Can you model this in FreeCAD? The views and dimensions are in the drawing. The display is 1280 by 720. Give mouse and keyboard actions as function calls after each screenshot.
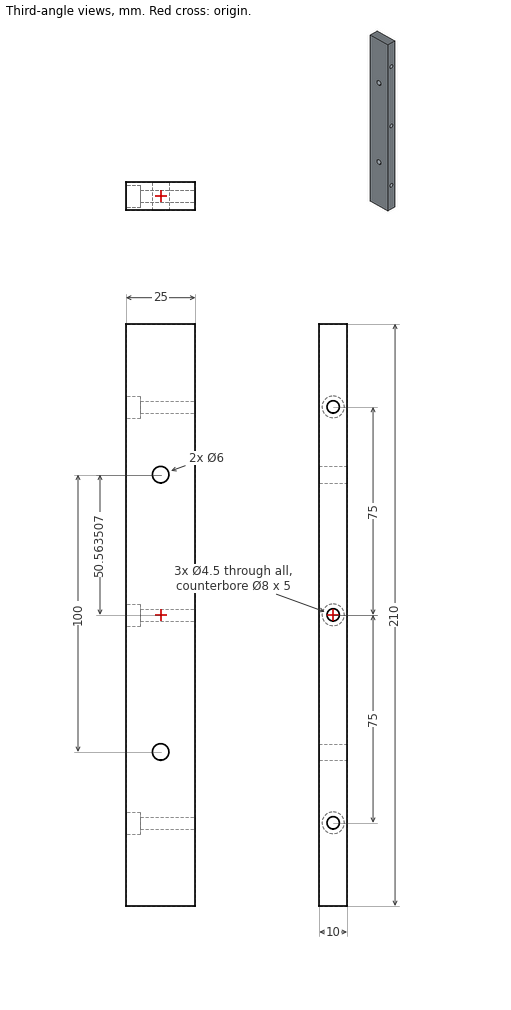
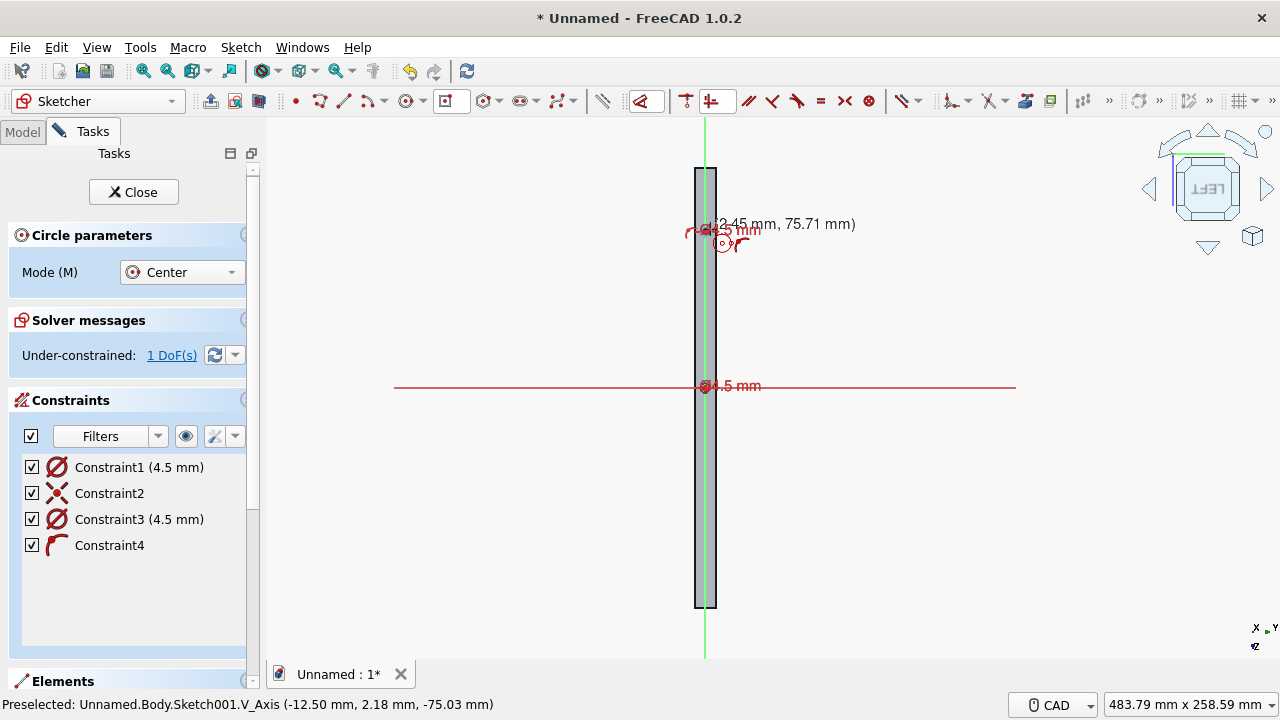
scroll(705, 545, up, 8)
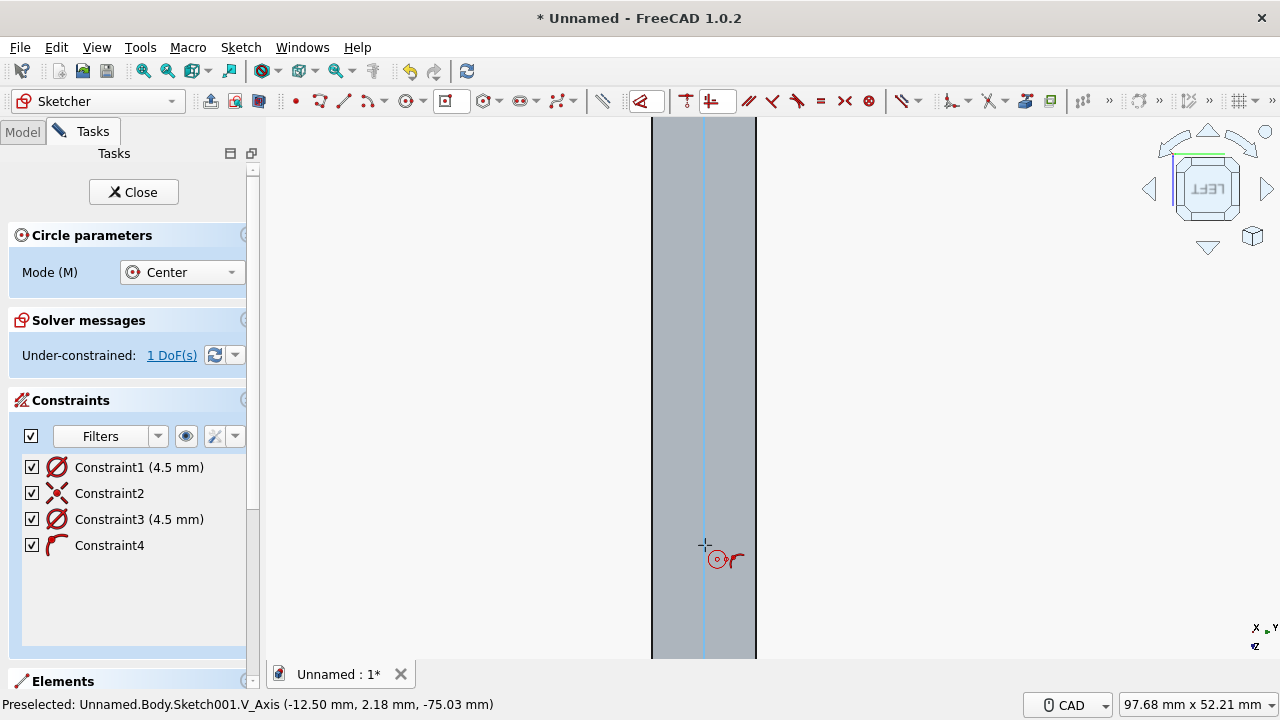
scroll(705, 546, down, 8)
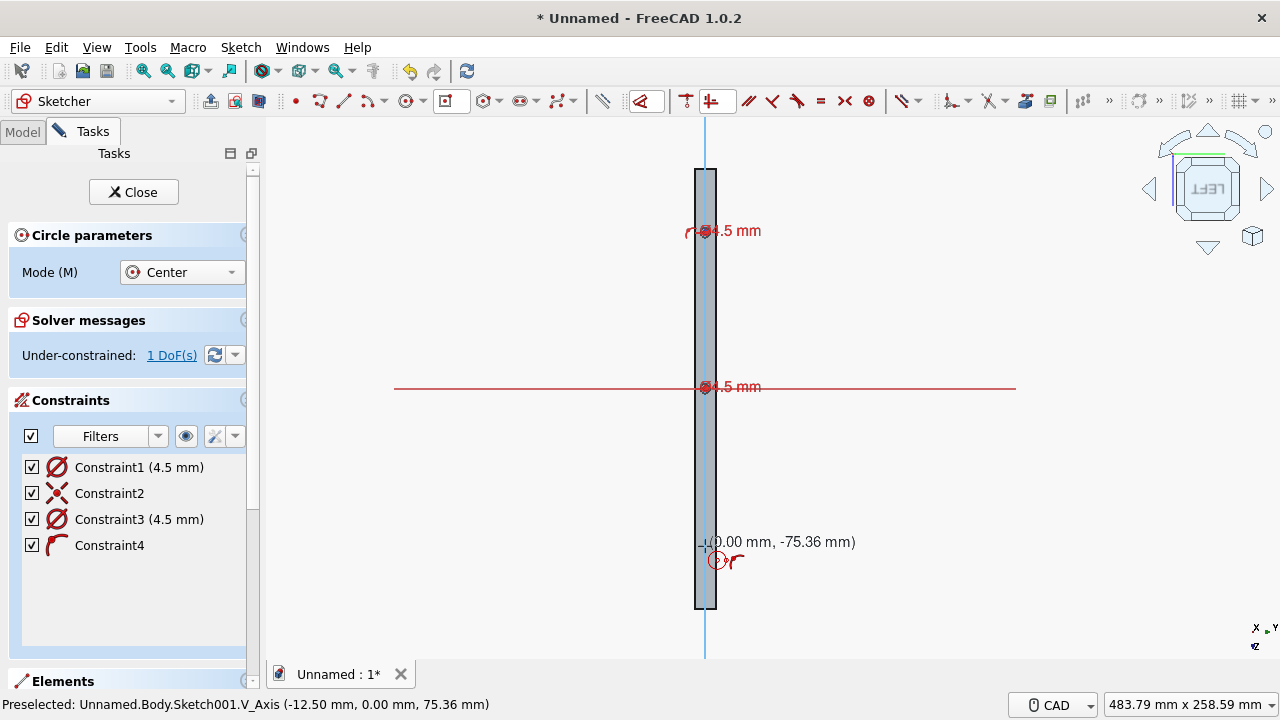
click(705, 546)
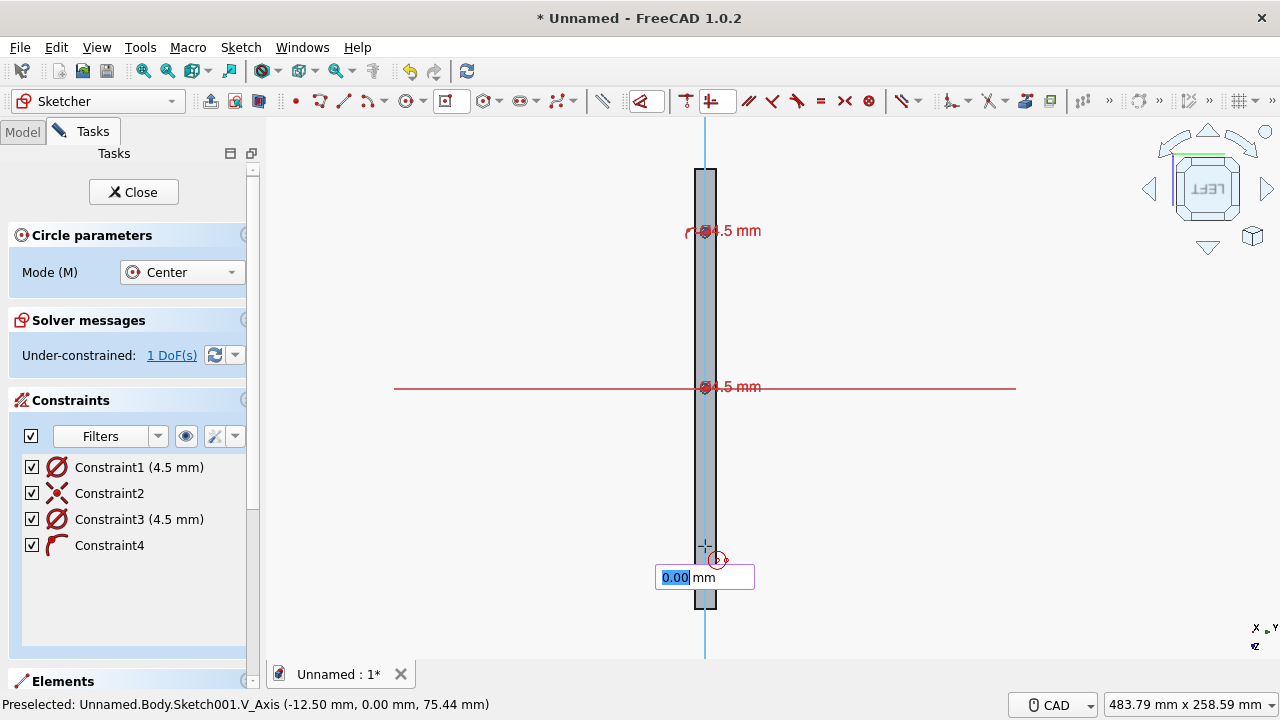
scroll(710, 544, up, 7)
move(707, 544)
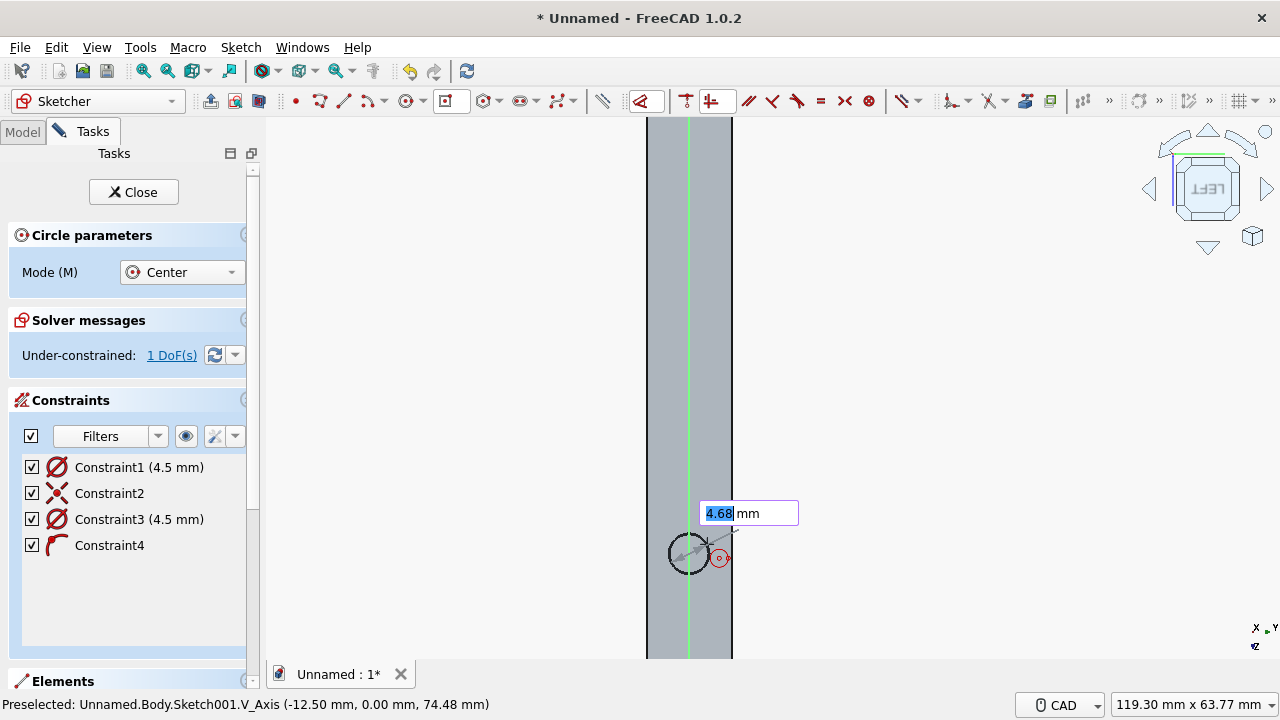
text(4.5)
key(Return)
key(Escape)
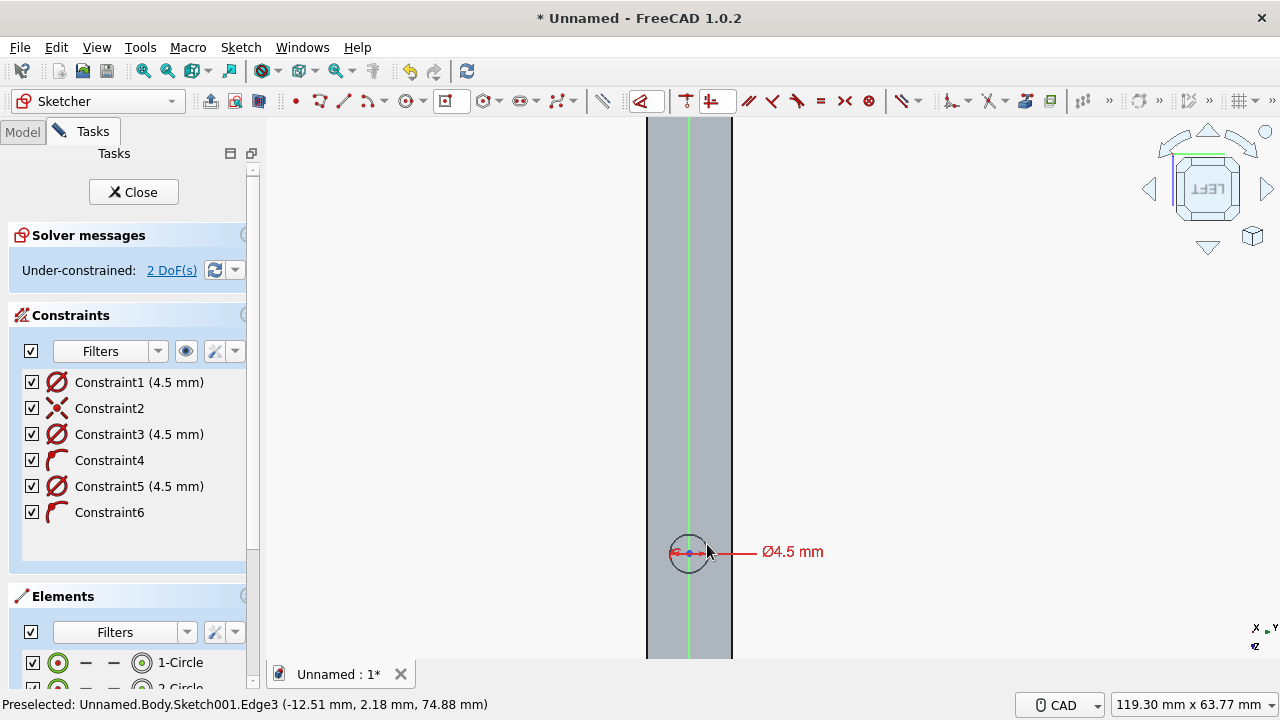
scroll(710, 544, down, 7)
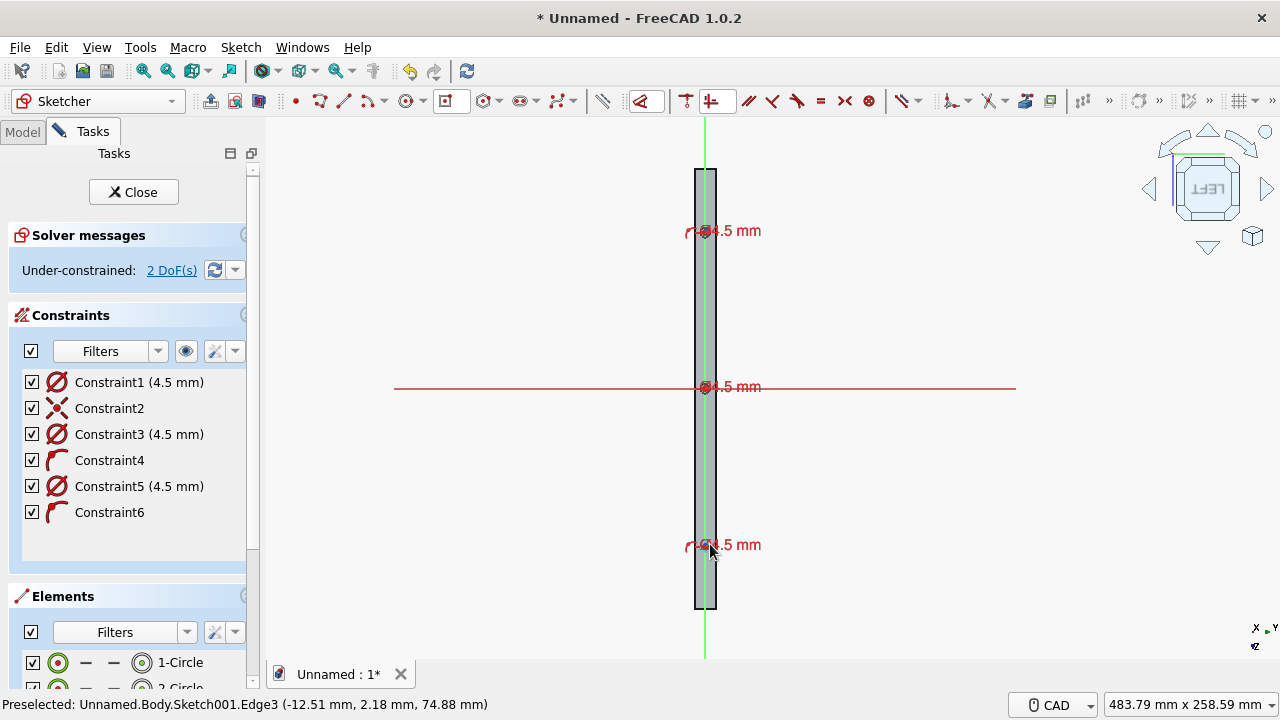
click(705, 233)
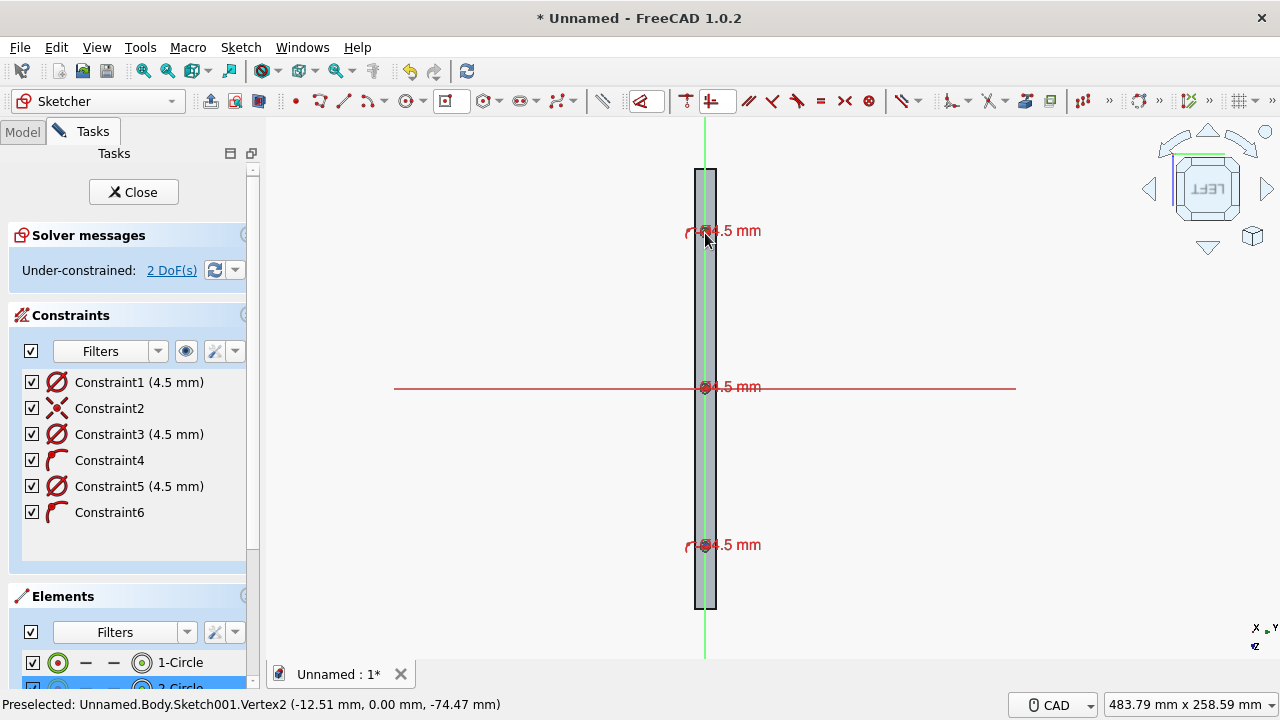
key(i)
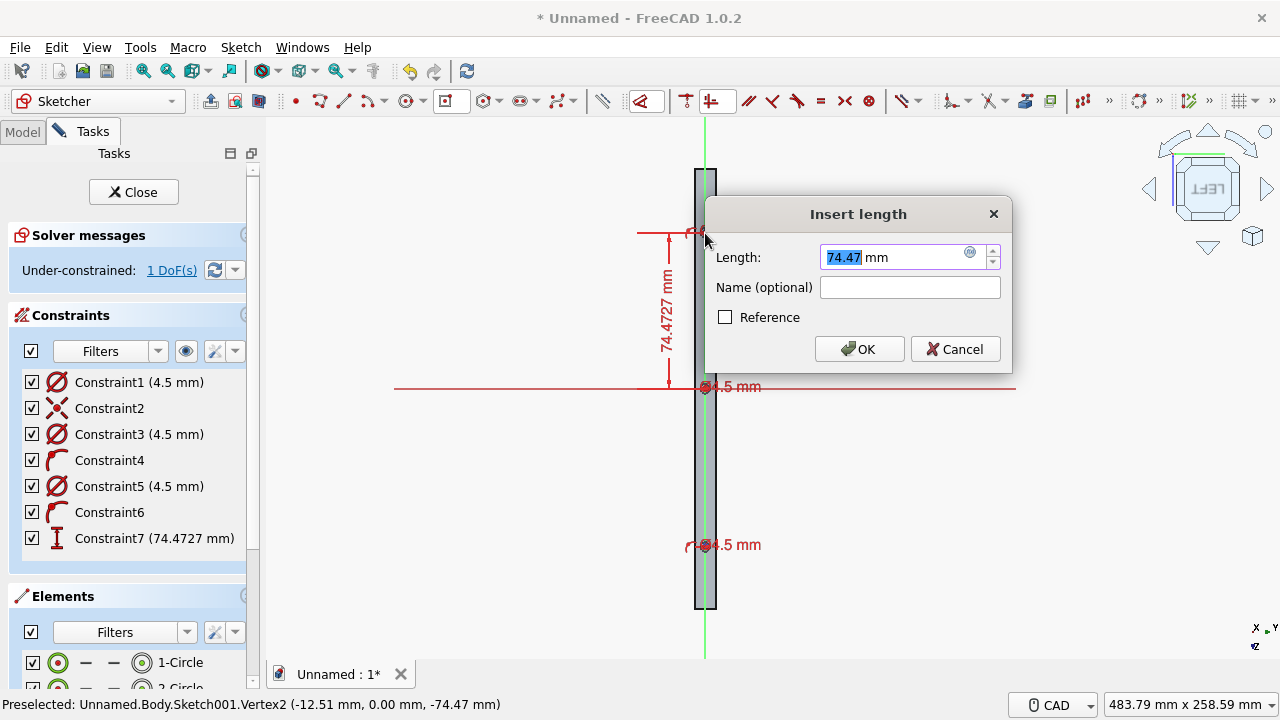
text(75)
key(Return)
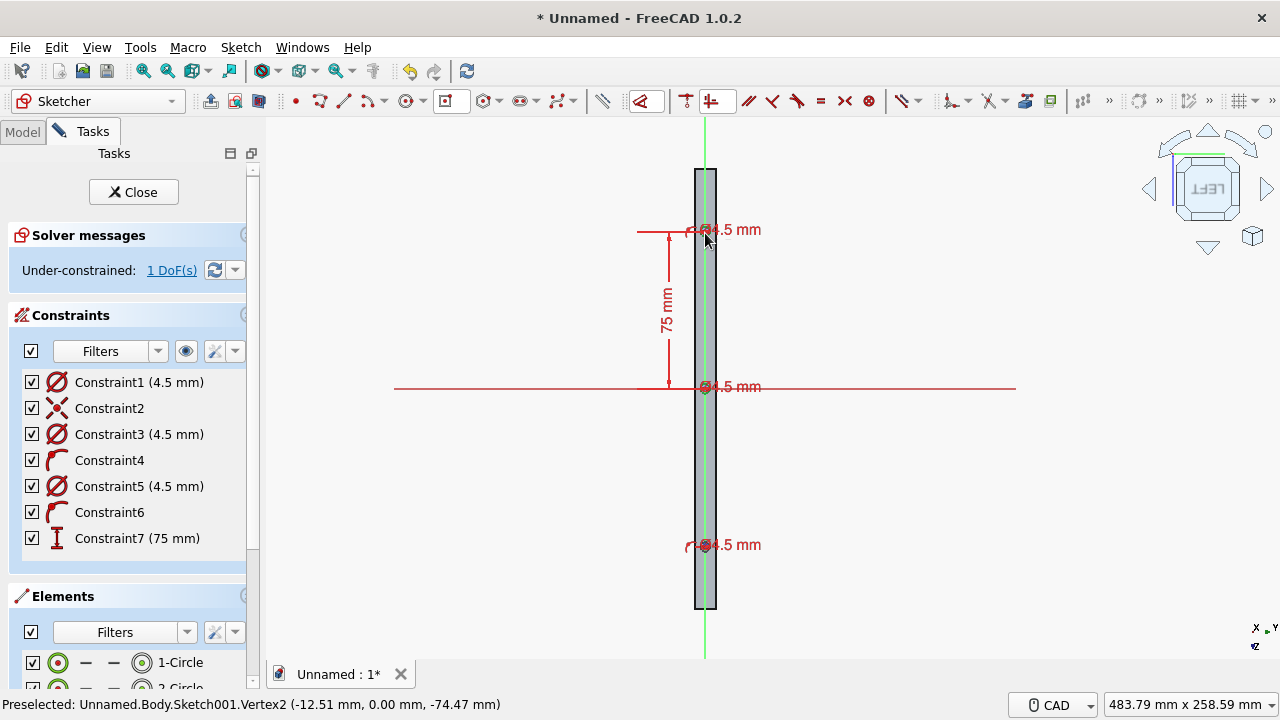
click(705, 547)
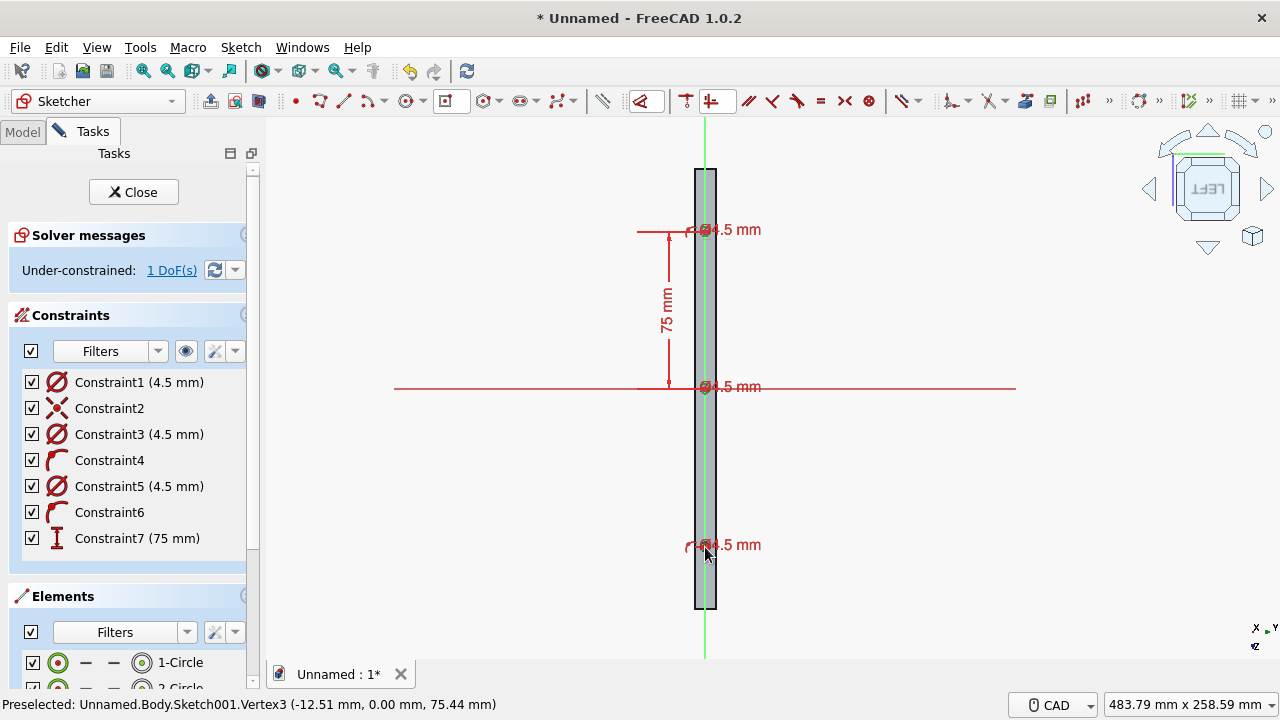
key(i)